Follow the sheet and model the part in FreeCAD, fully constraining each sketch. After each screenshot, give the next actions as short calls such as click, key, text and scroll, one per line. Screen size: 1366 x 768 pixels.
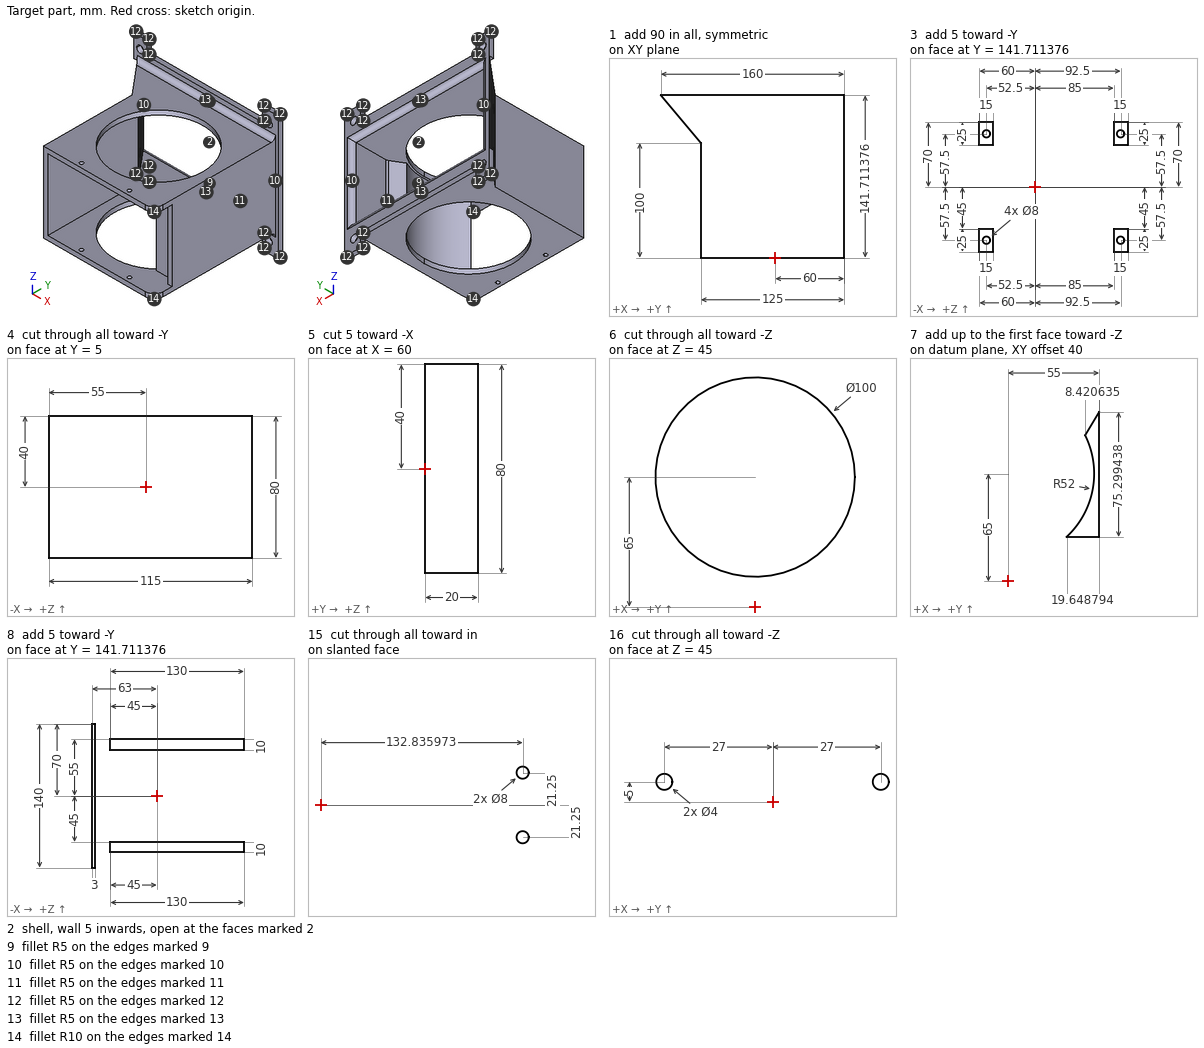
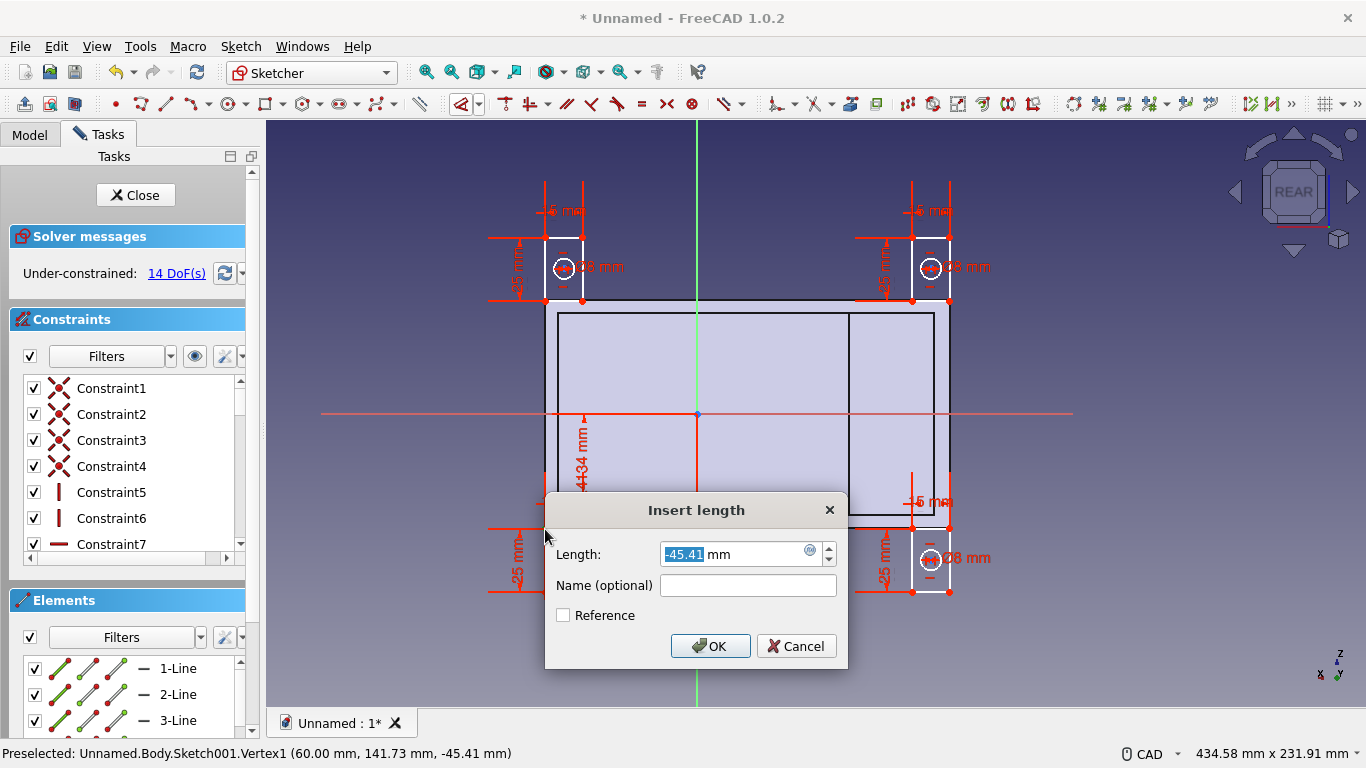
text(-45)
key(Return)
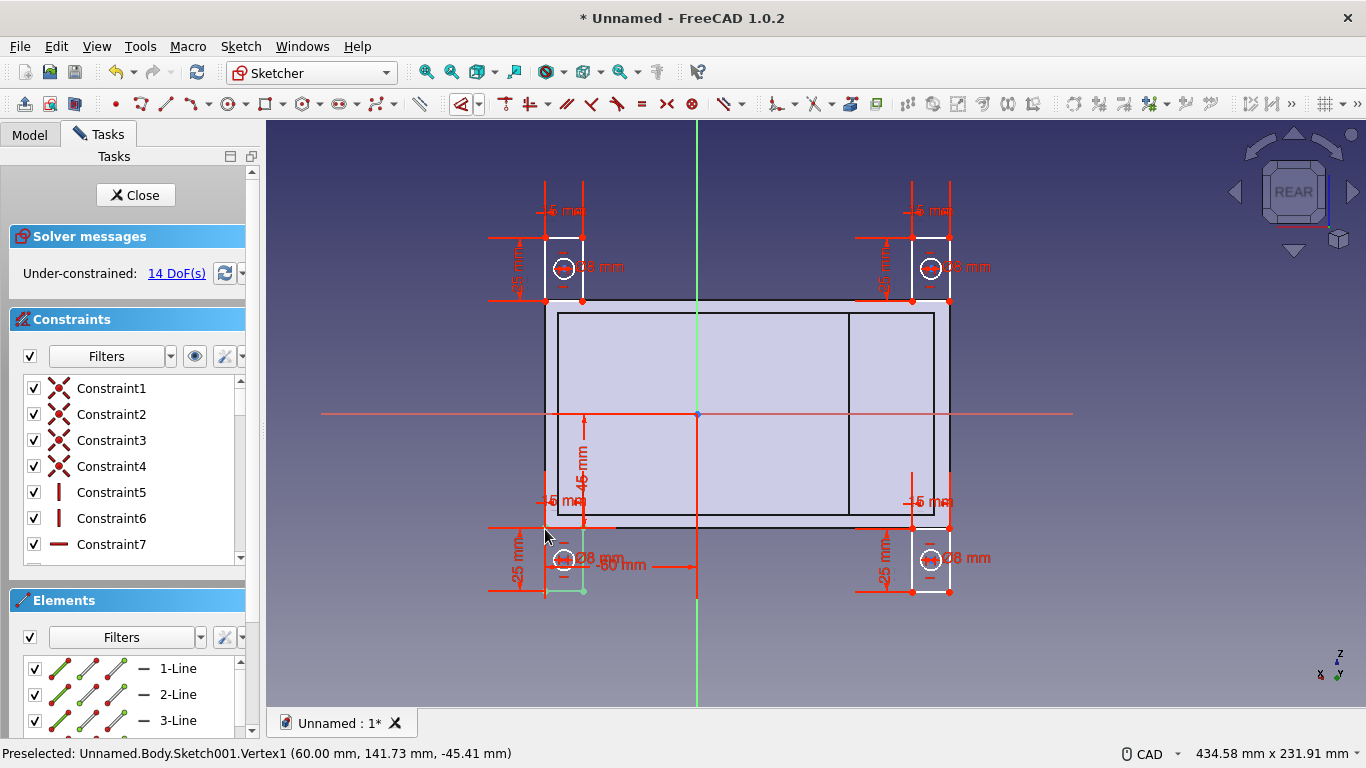
click(912, 238)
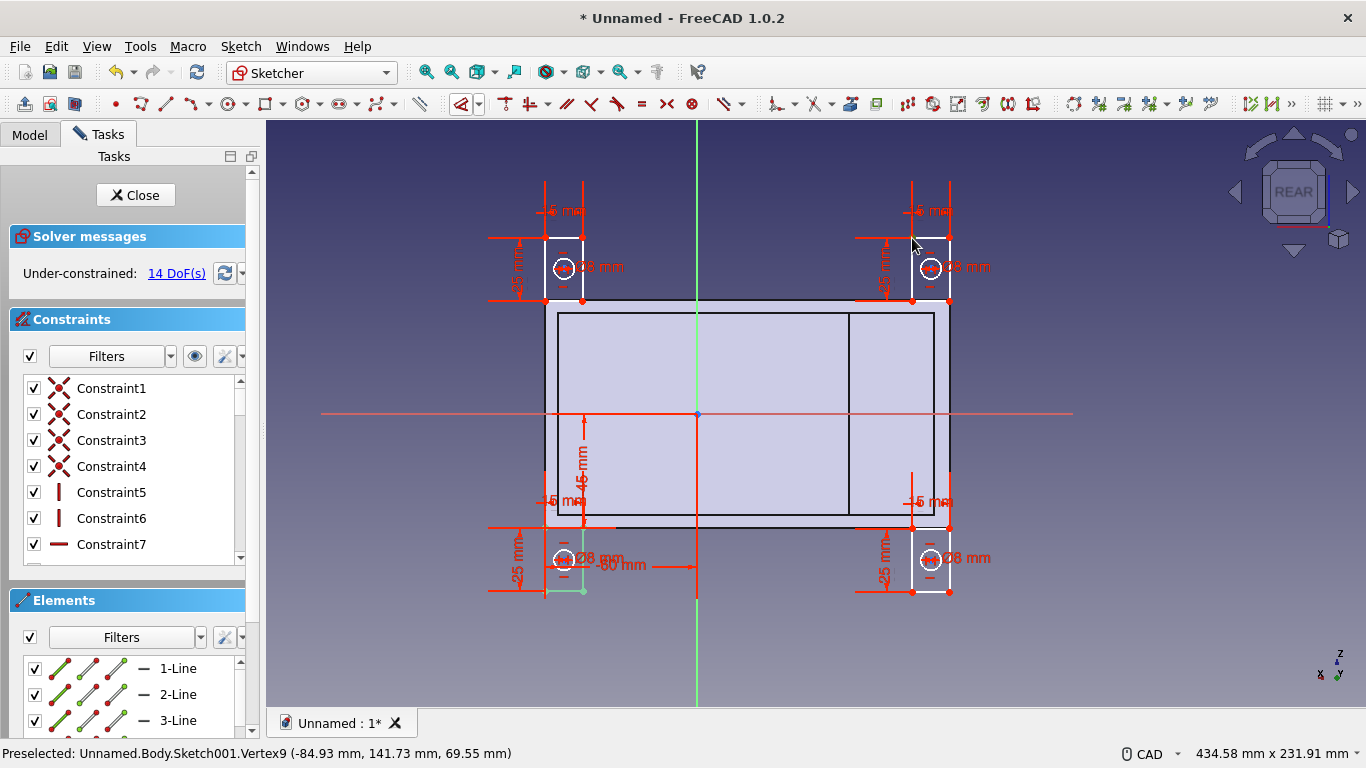
key(l)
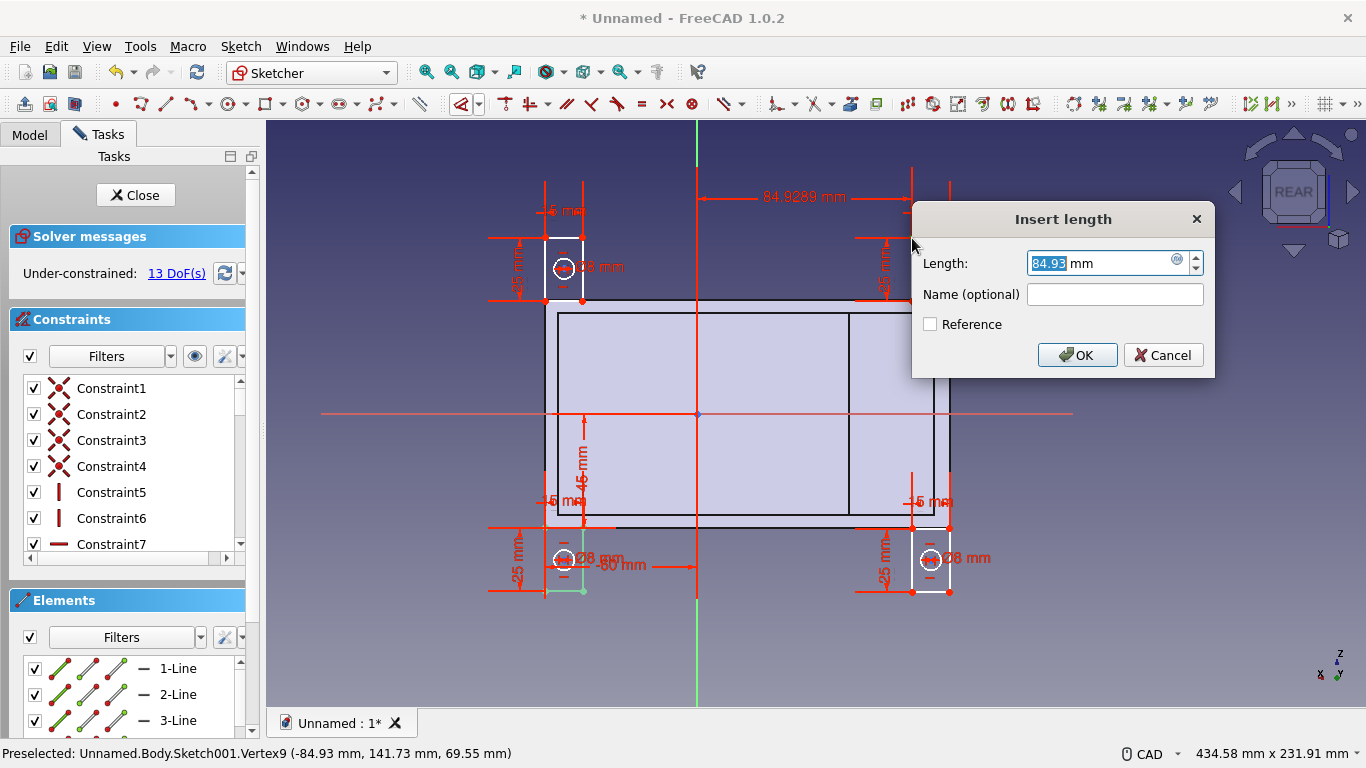
text(85)
key(Return)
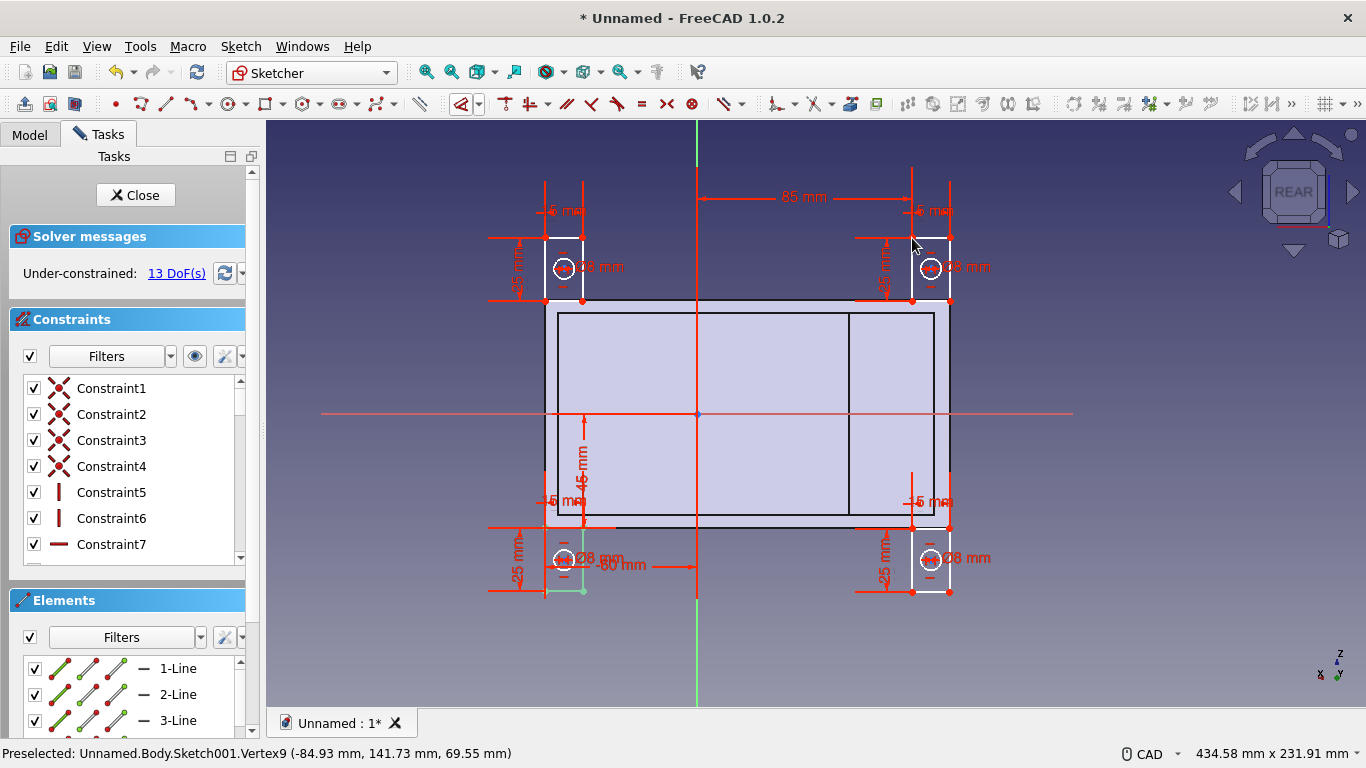
click(912, 238)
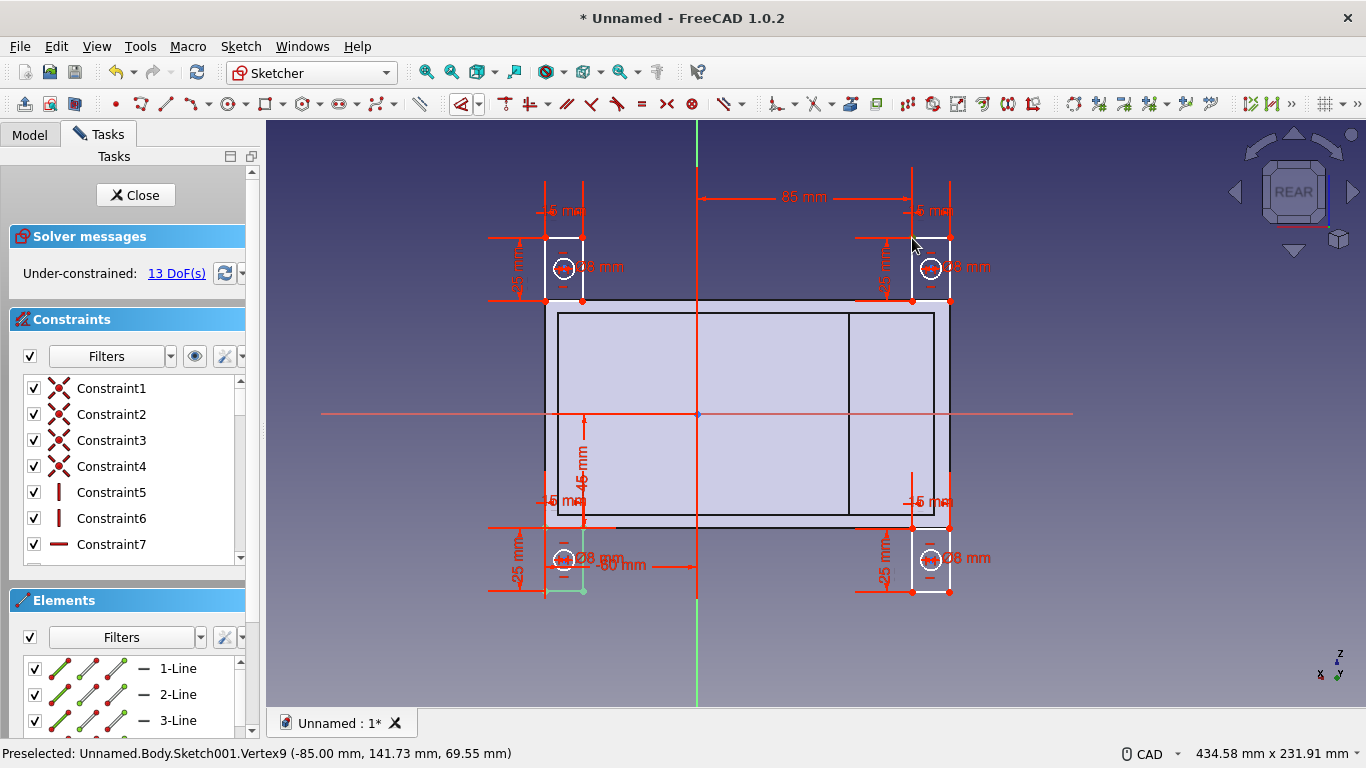
key(i)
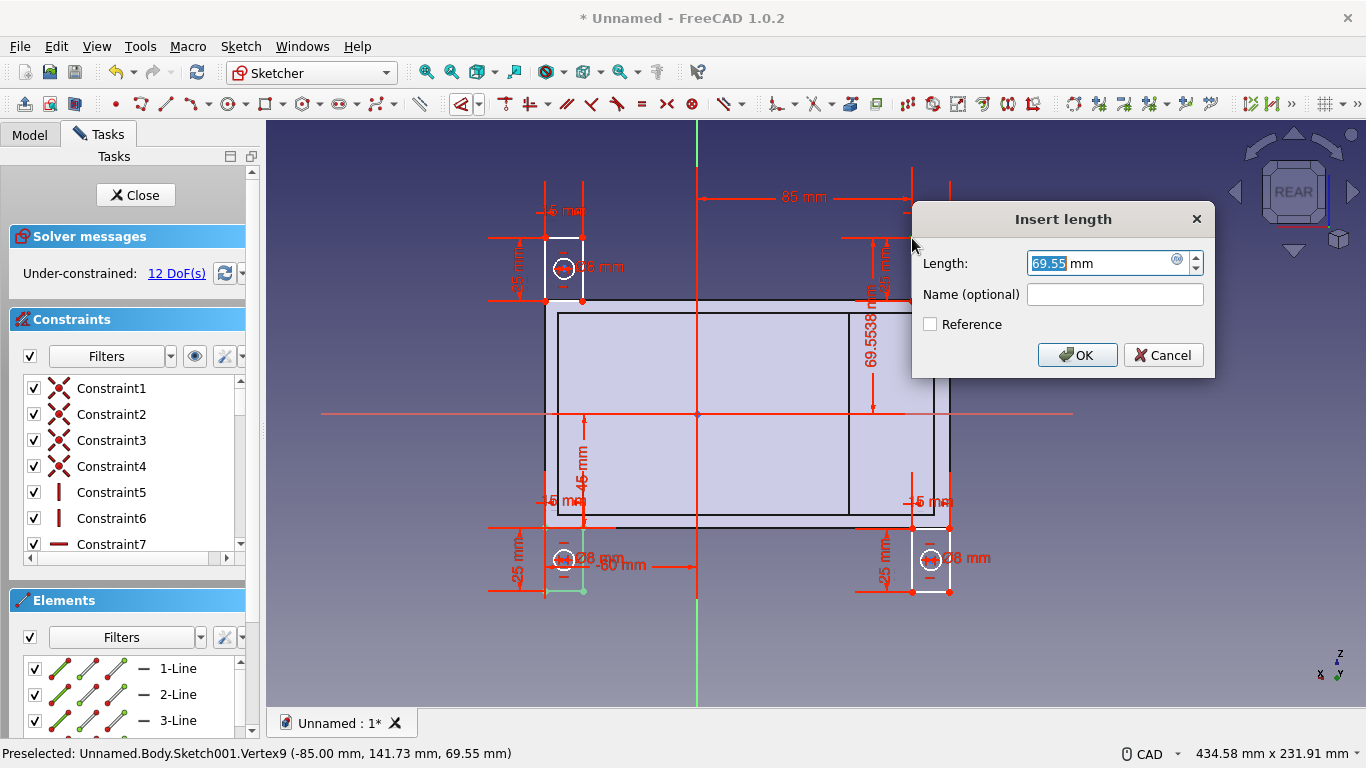
text(70)
key(Return)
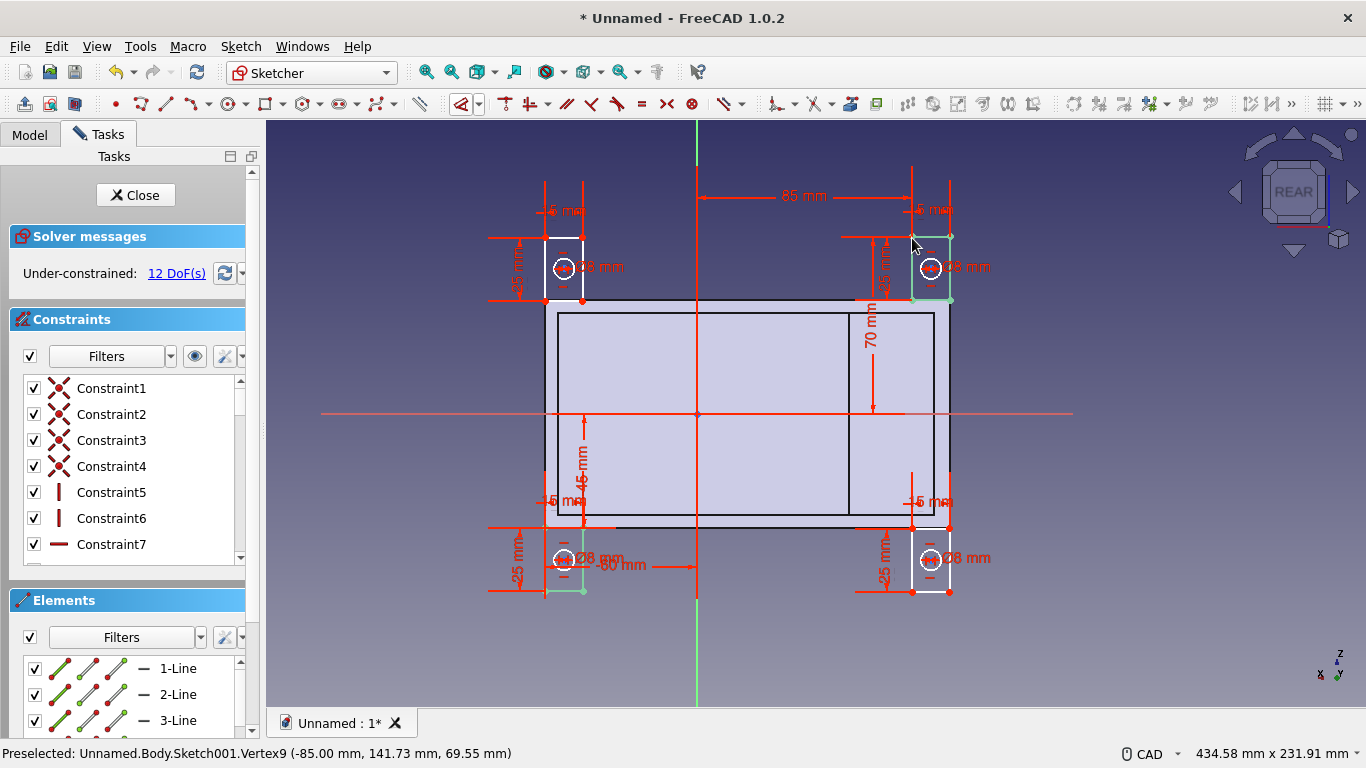
click(545, 238)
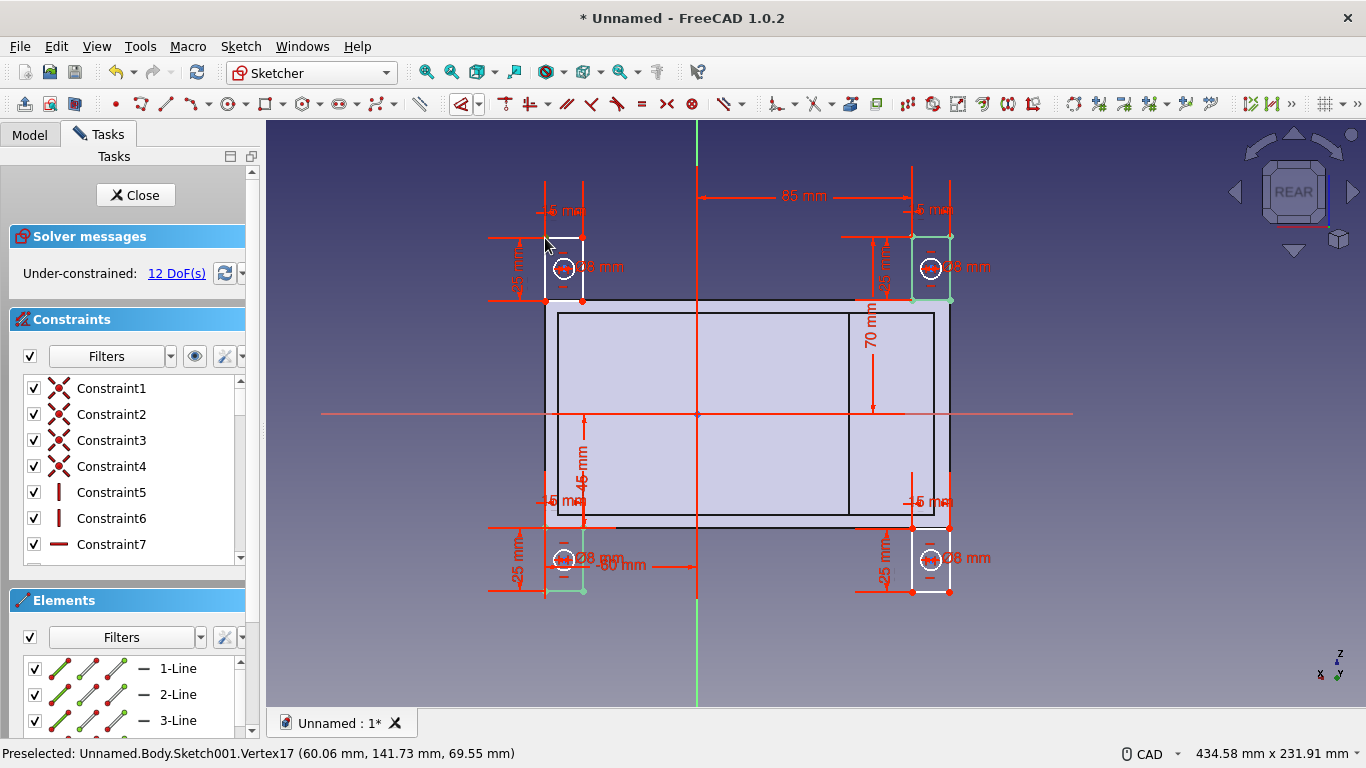
click(478, 104)